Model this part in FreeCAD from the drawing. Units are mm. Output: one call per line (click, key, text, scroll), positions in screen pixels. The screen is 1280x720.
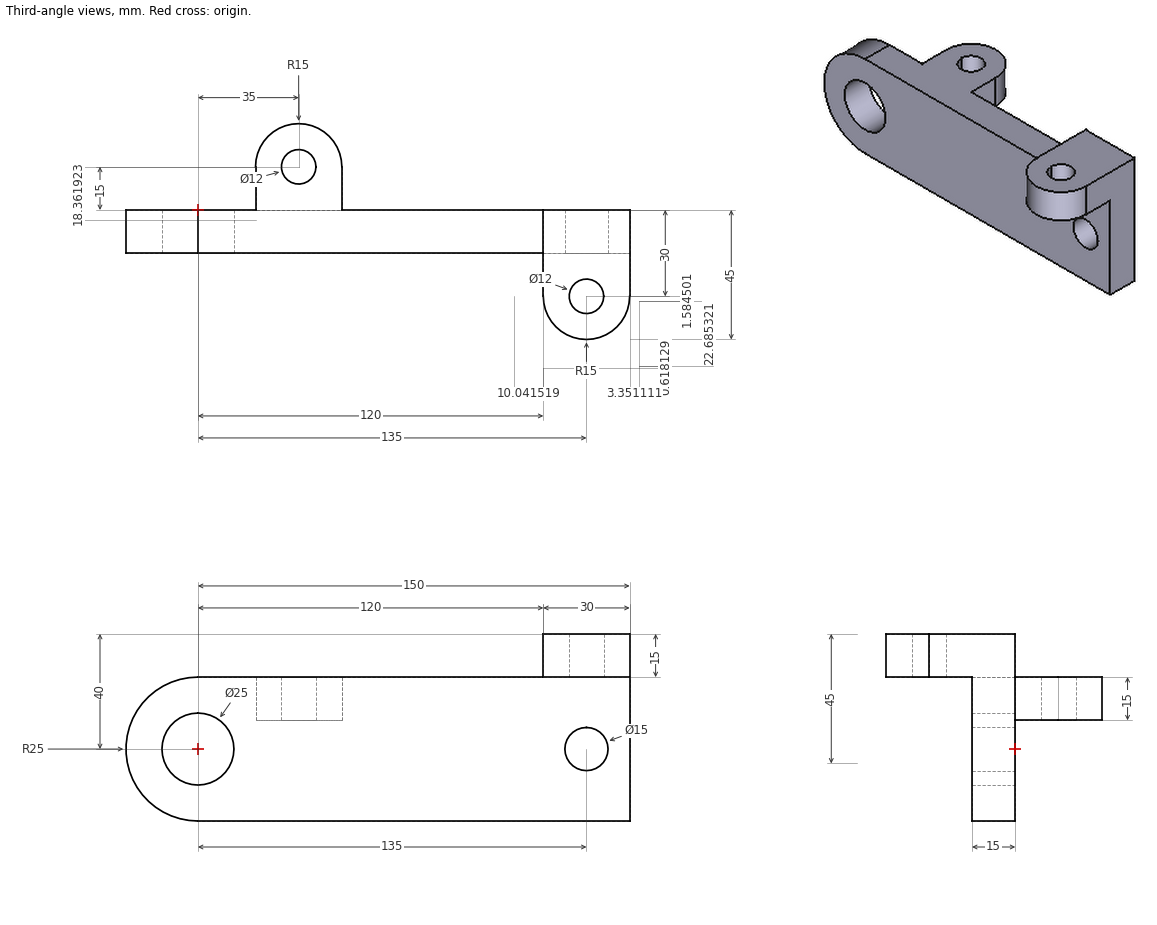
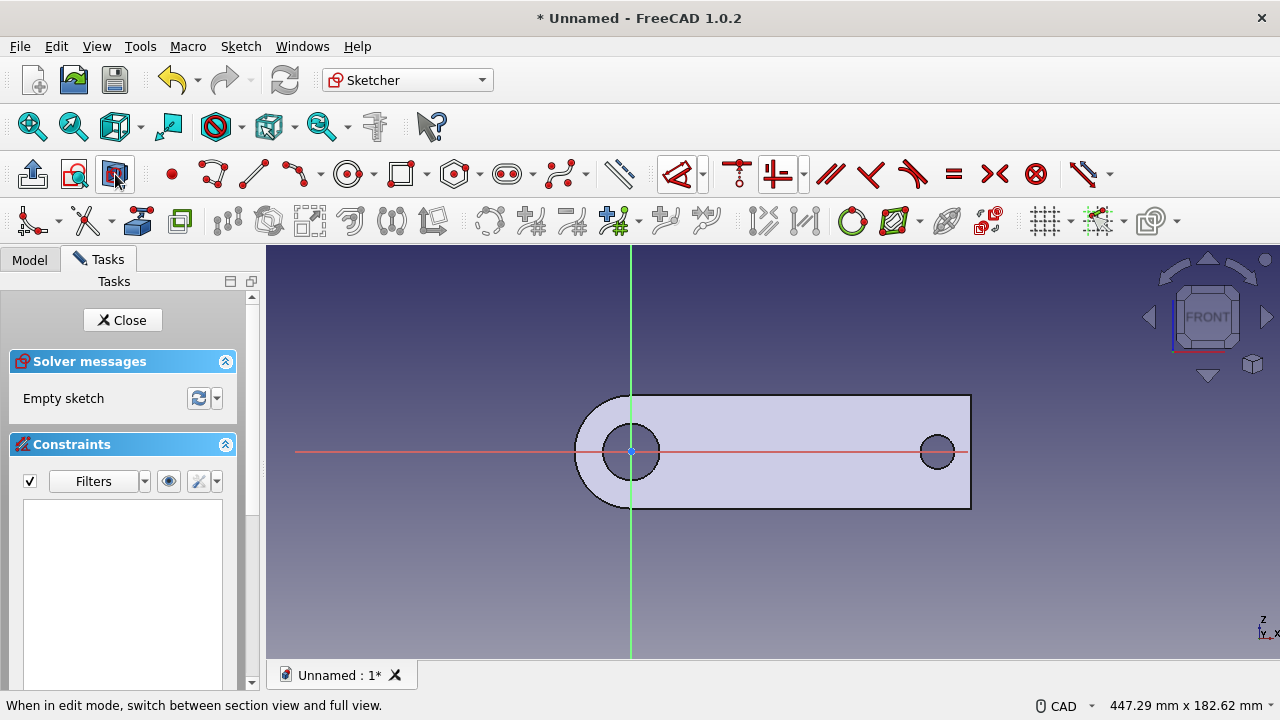
scroll(974, 367, up, 10)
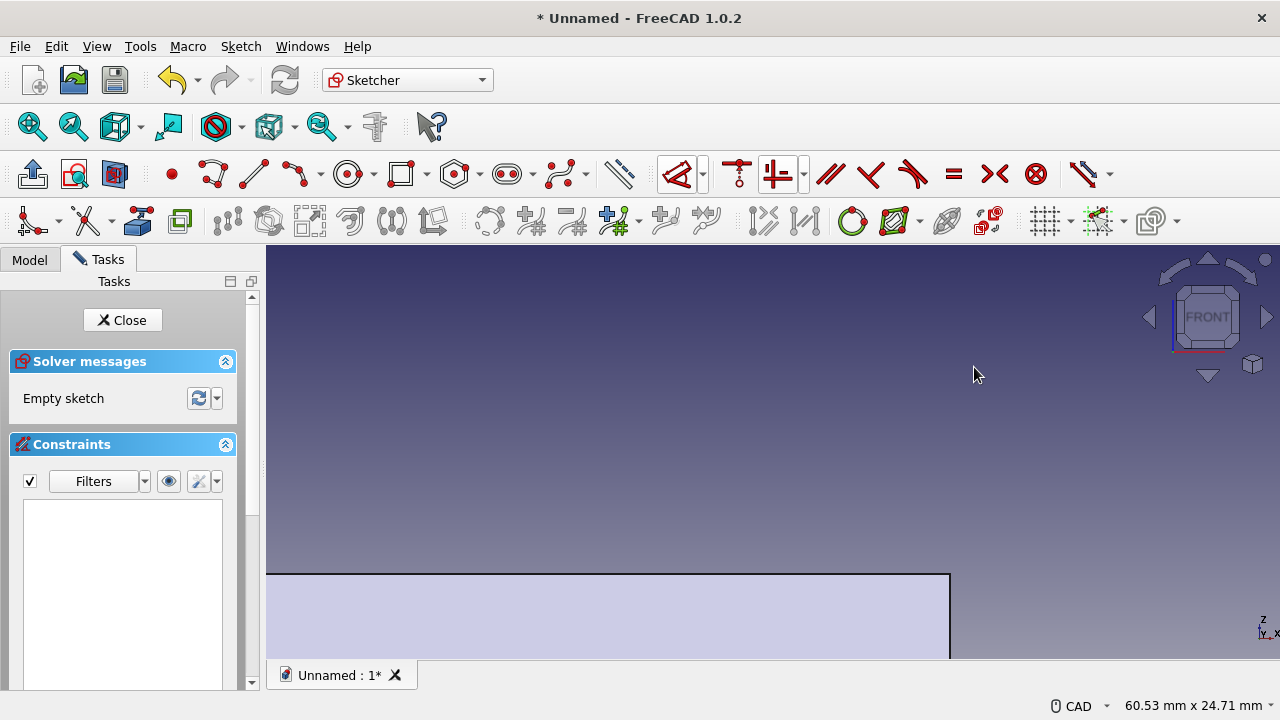
click(400, 174)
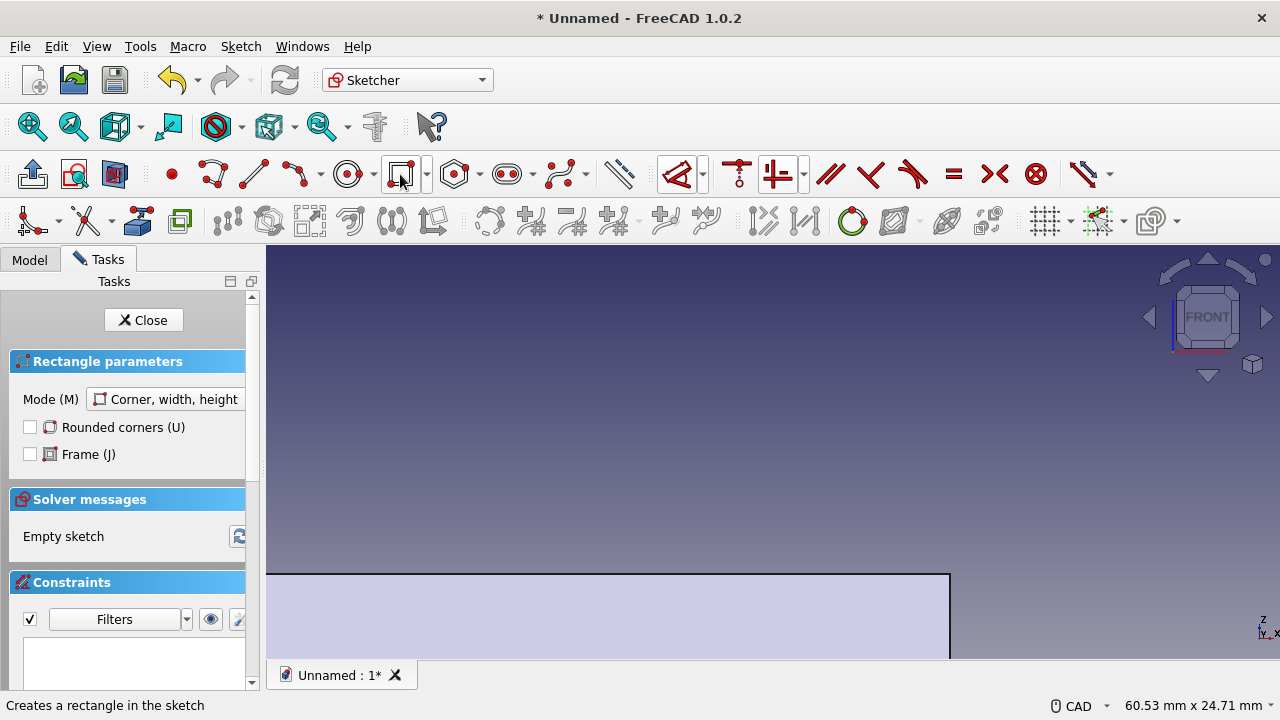
click(448, 323)
click(950, 574)
key(Escape)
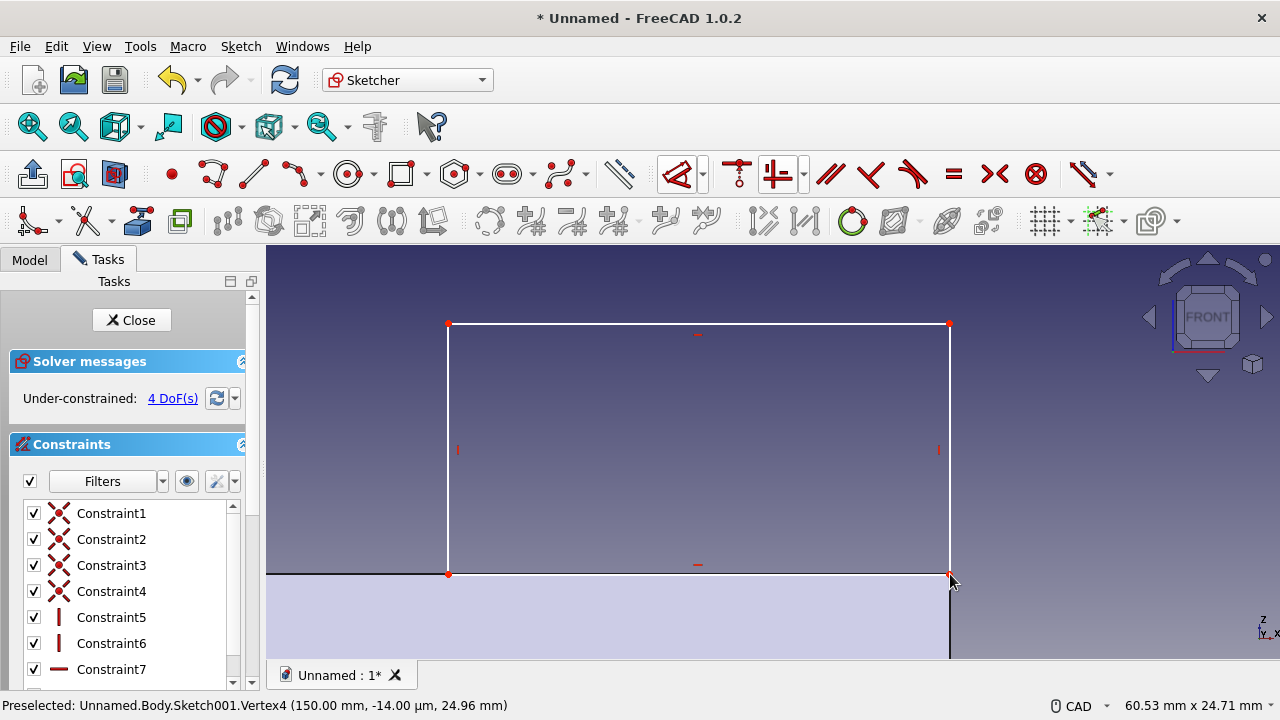
click(448, 399)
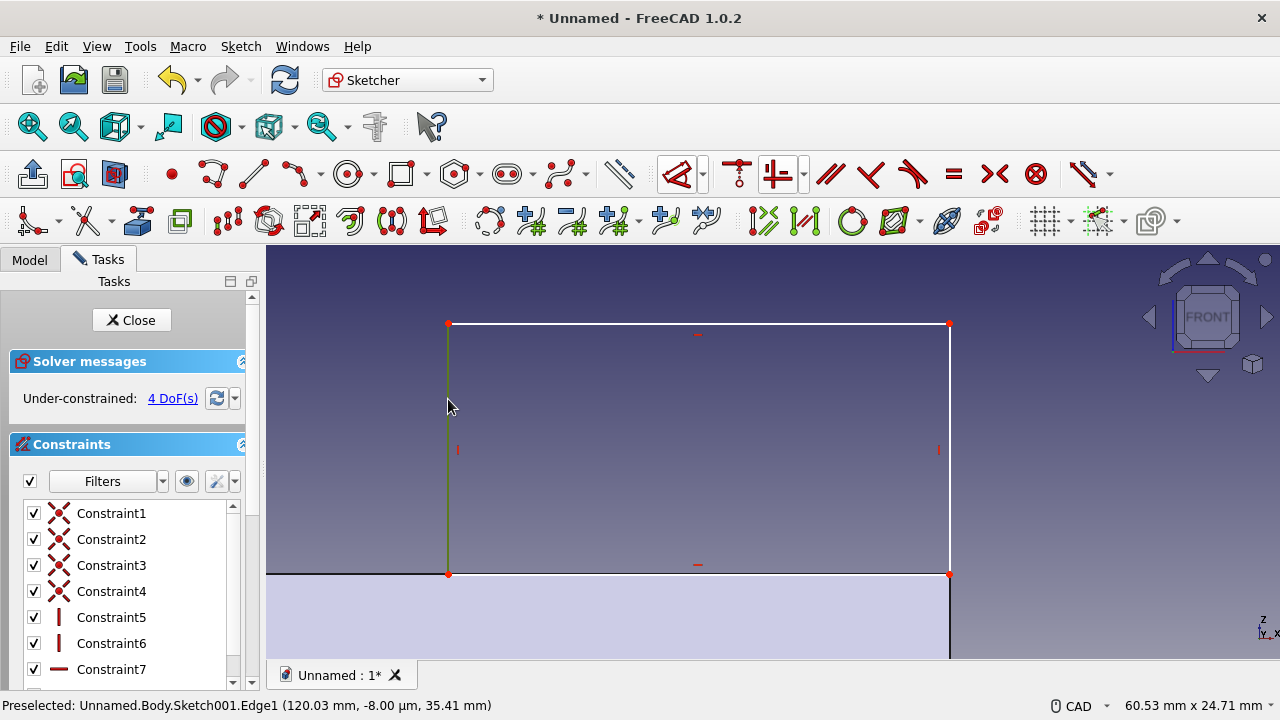
key(i)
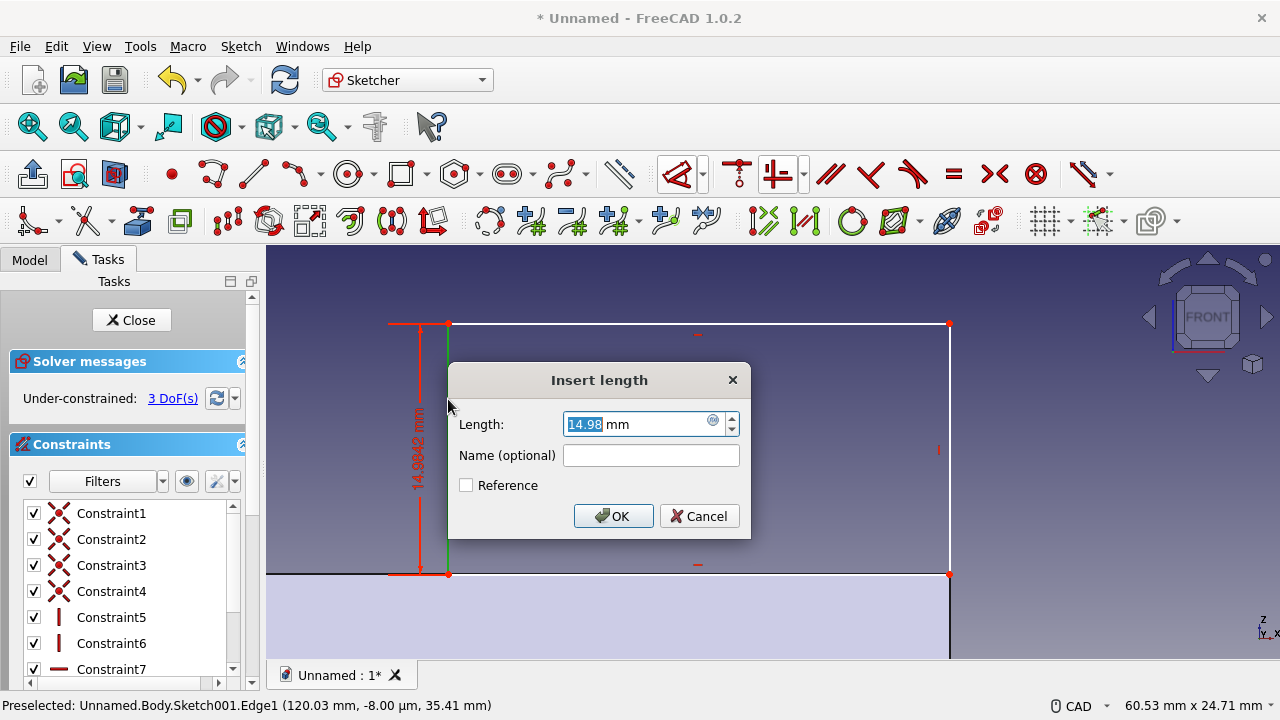
text(15)
key(Return)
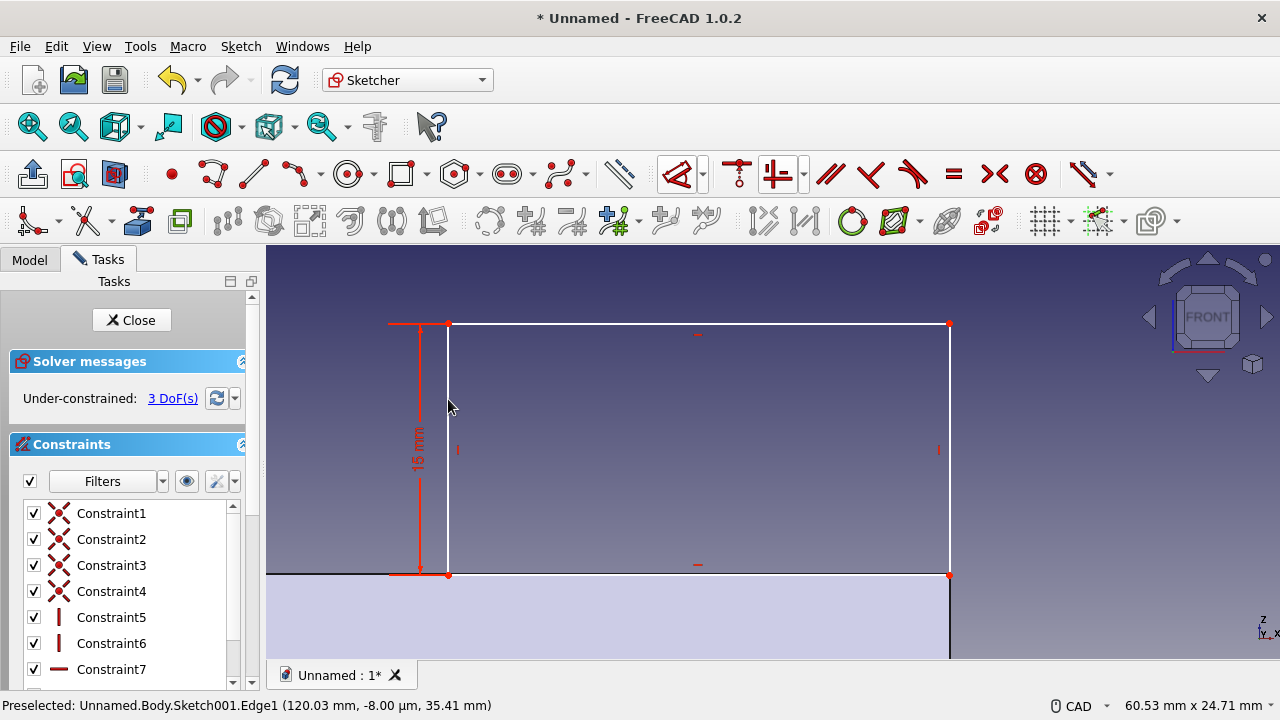
click(599, 575)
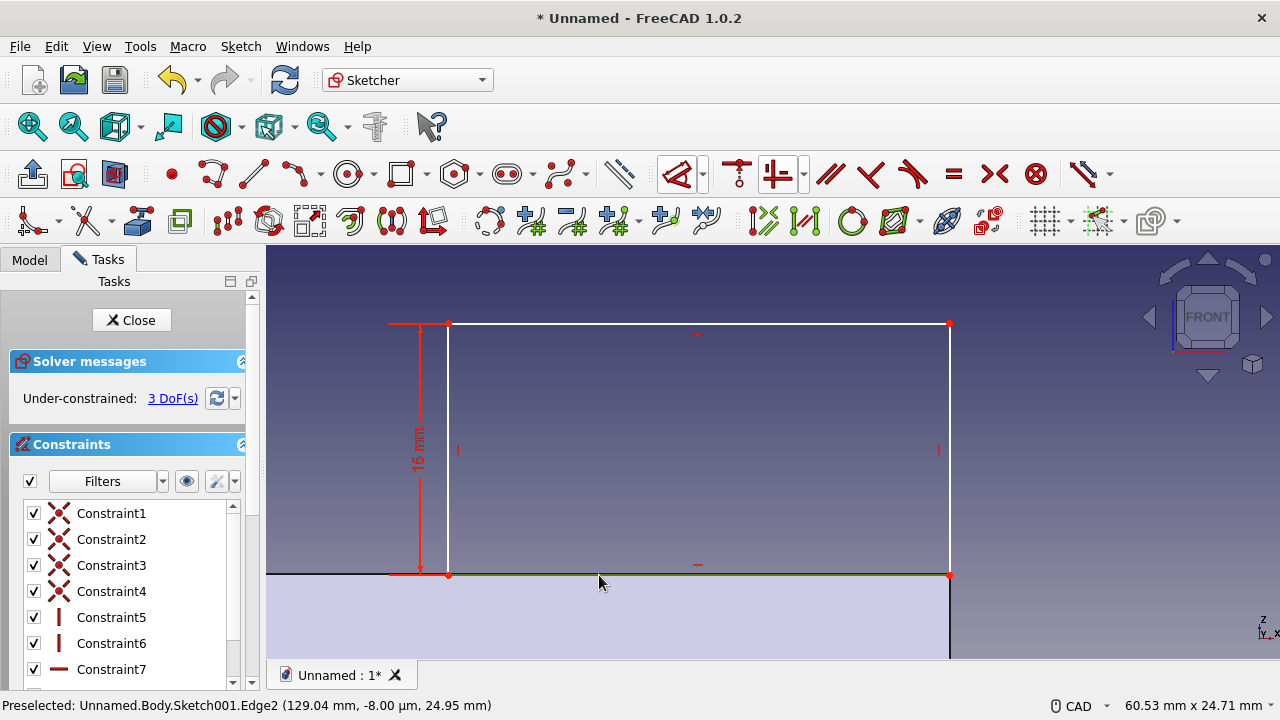
click(702, 174)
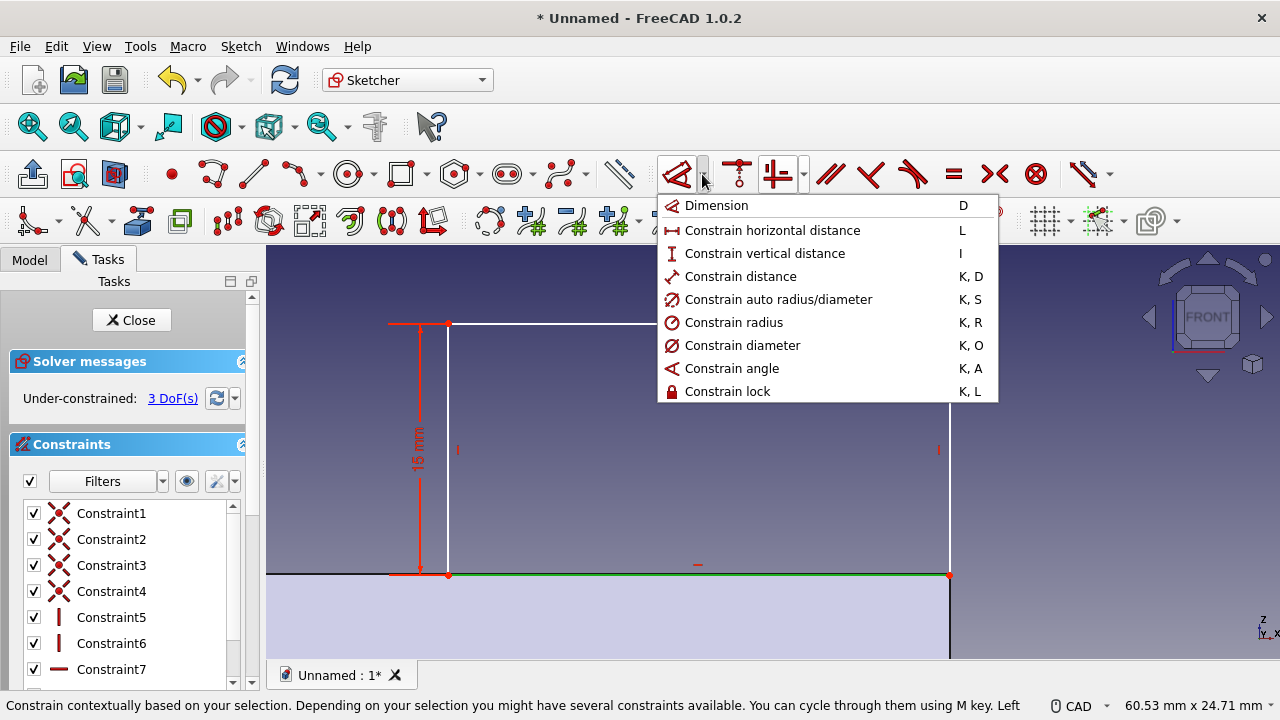
click(828, 230)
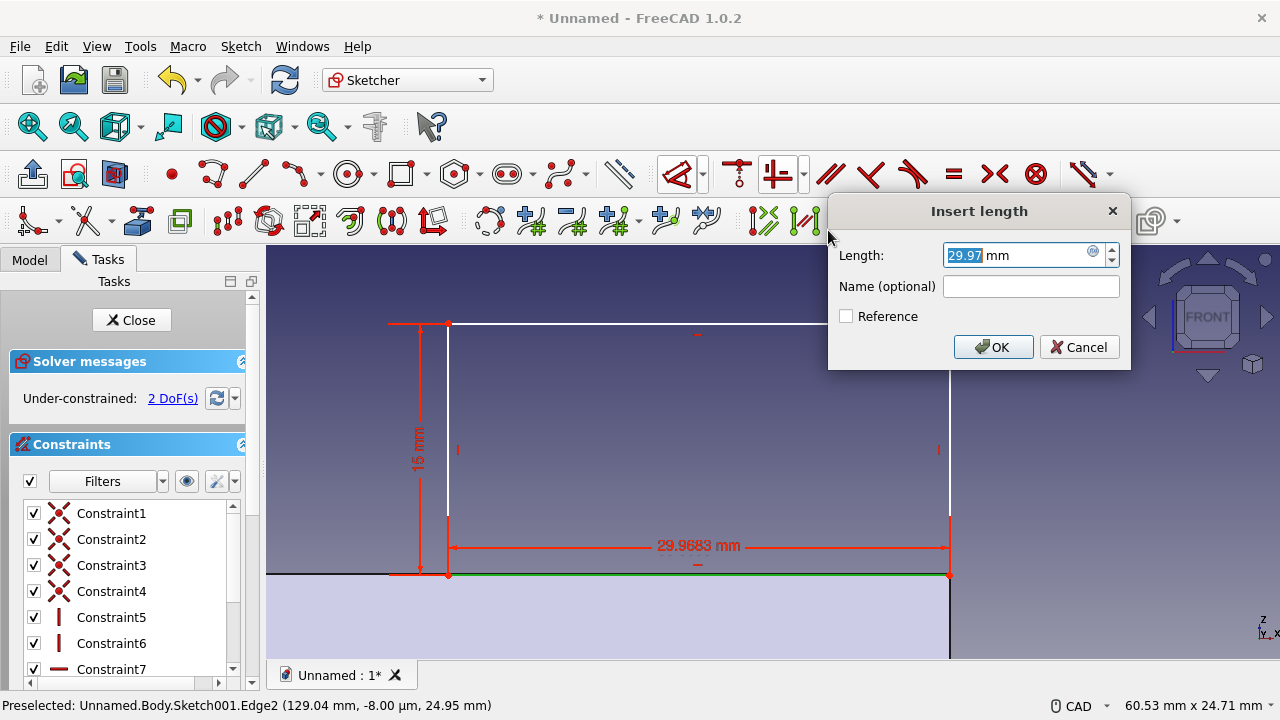
text(30)
key(Return)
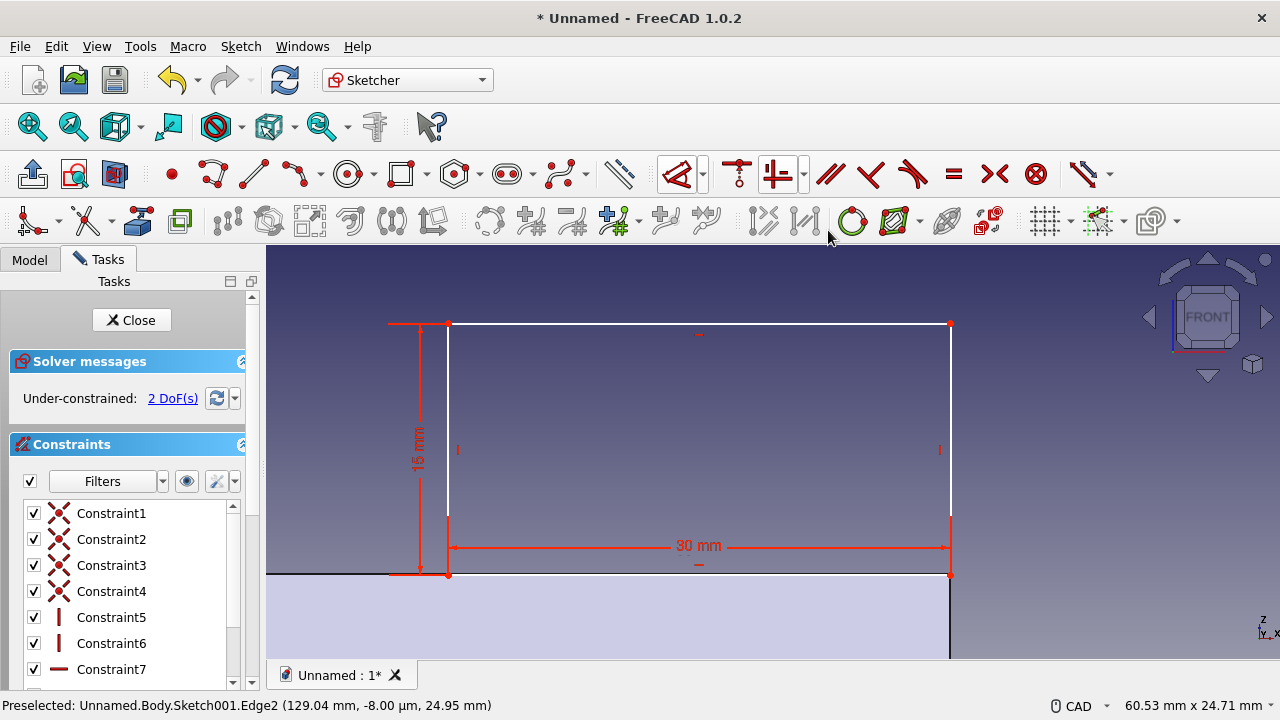
click(448, 324)